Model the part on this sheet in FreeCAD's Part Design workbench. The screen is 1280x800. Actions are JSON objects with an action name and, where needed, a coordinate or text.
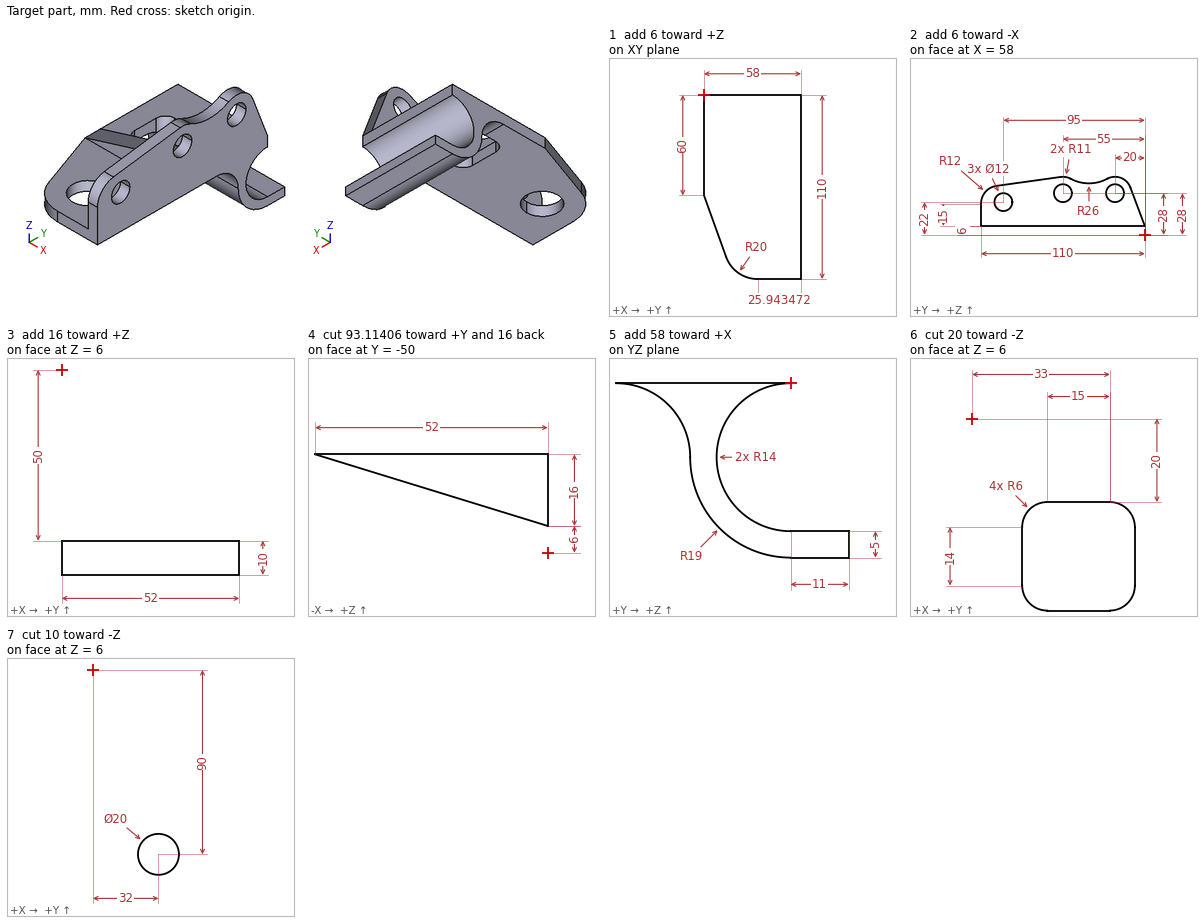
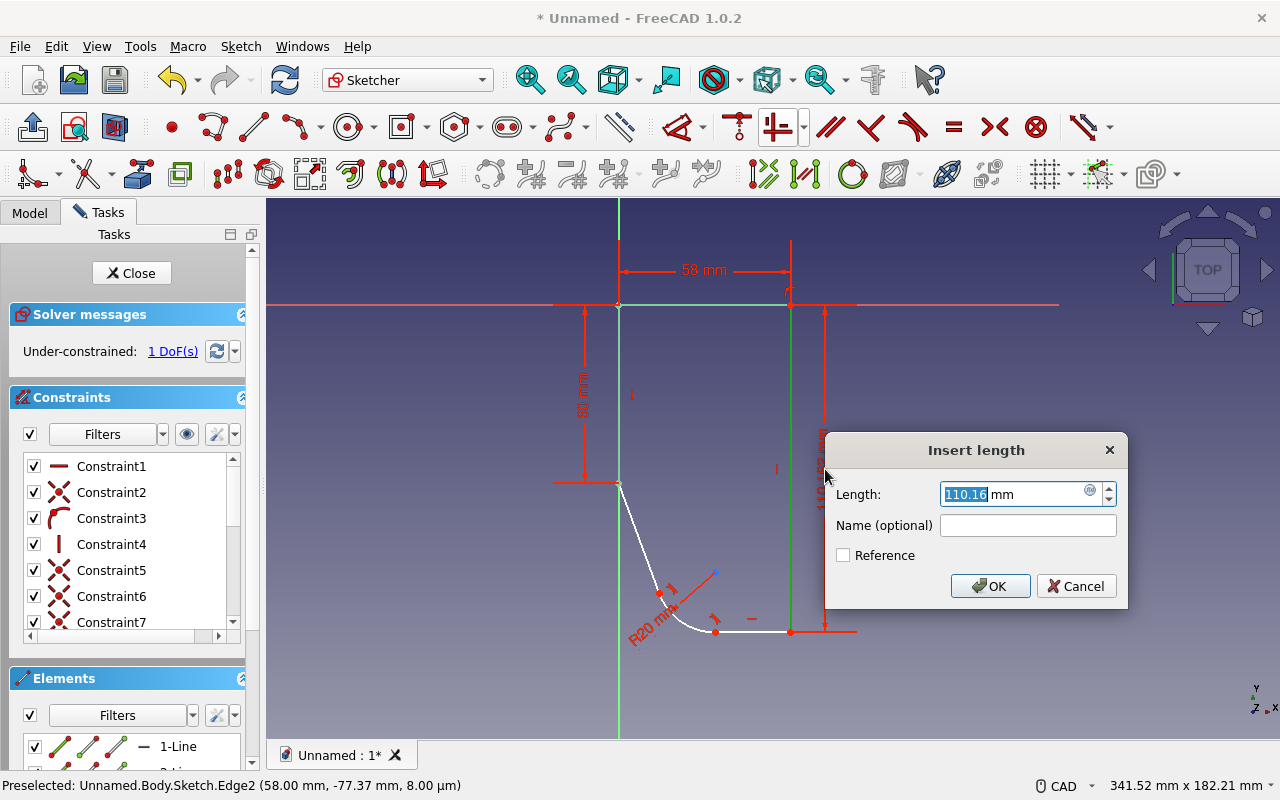
{"action": "type", "text": "110"}
{"action": "key", "text": "Return"}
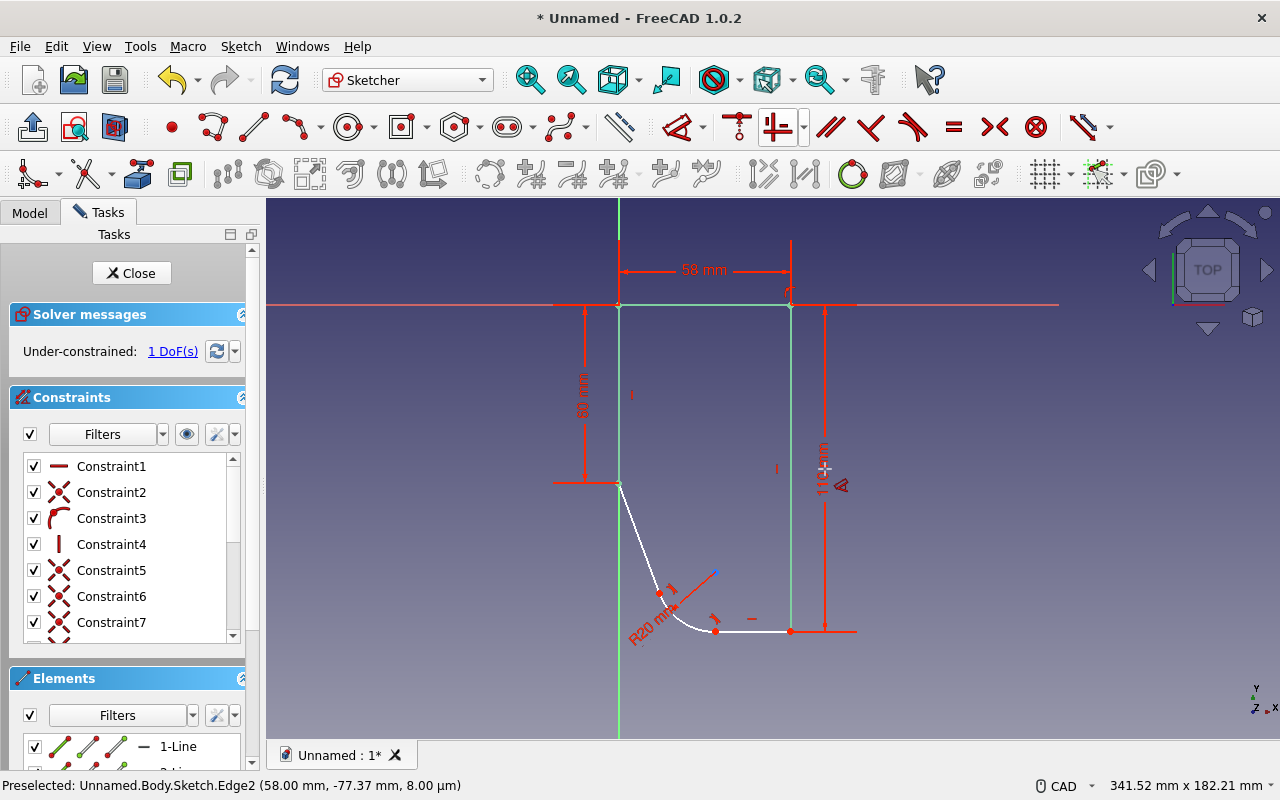
{"action": "left_click", "coordinate": [738, 632]}
{"action": "left_click", "coordinate": [753, 666]}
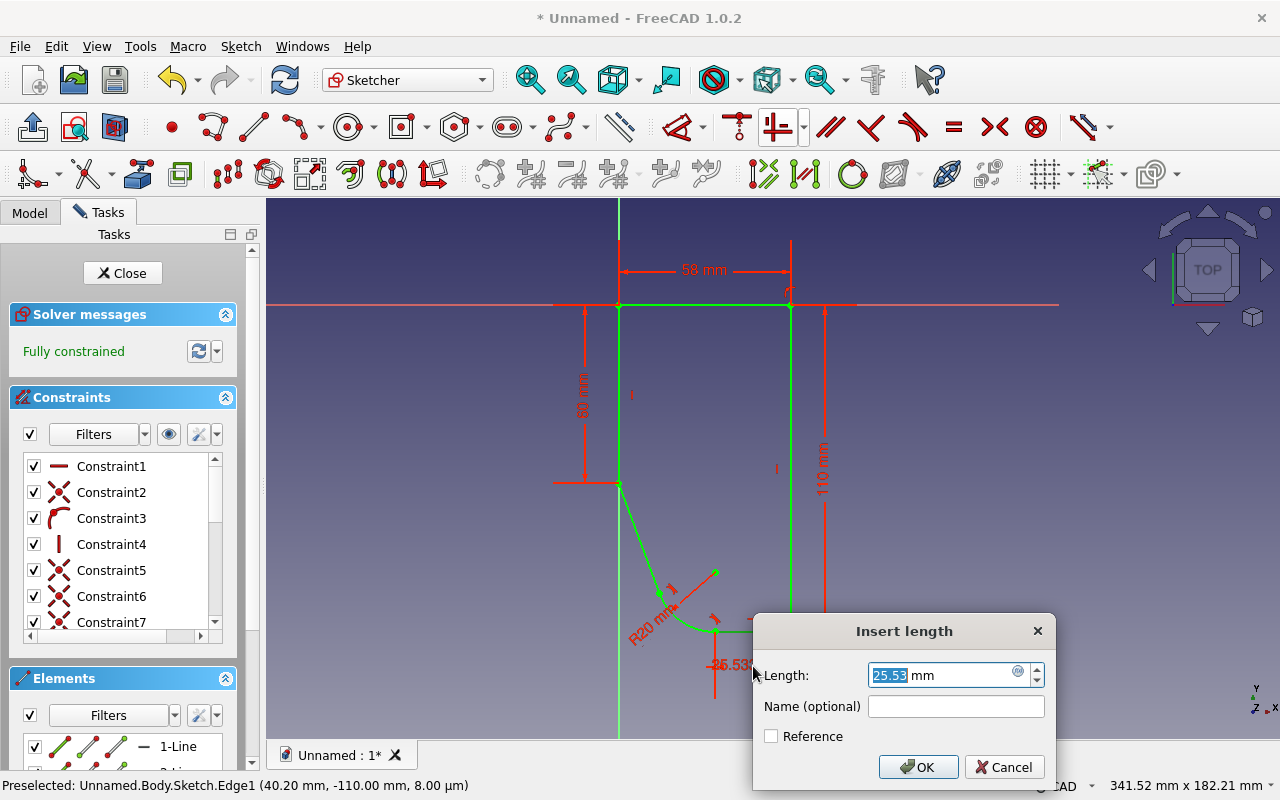
{"action": "type", "text": "25.943472"}
{"action": "key", "text": "Return"}
{"action": "key", "text": "Escape"}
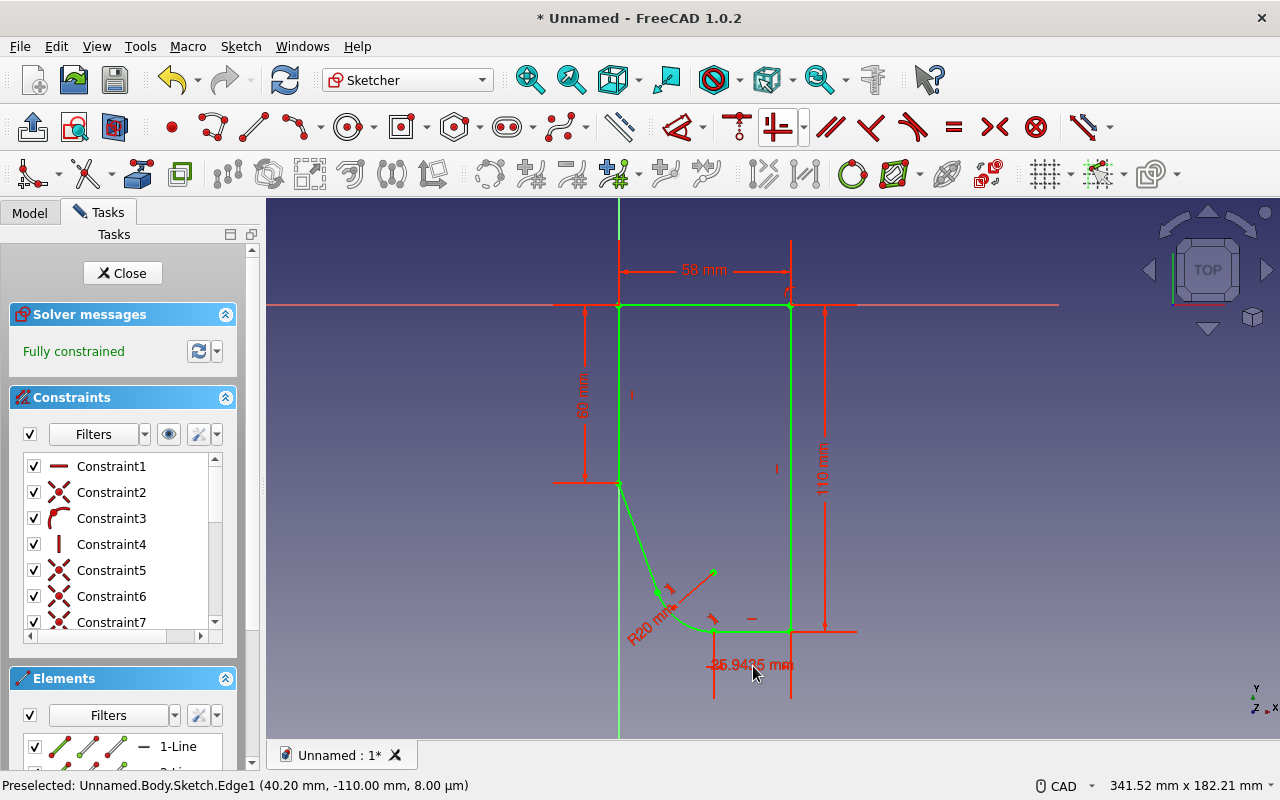
{"action": "left_click", "coordinate": [123, 273]}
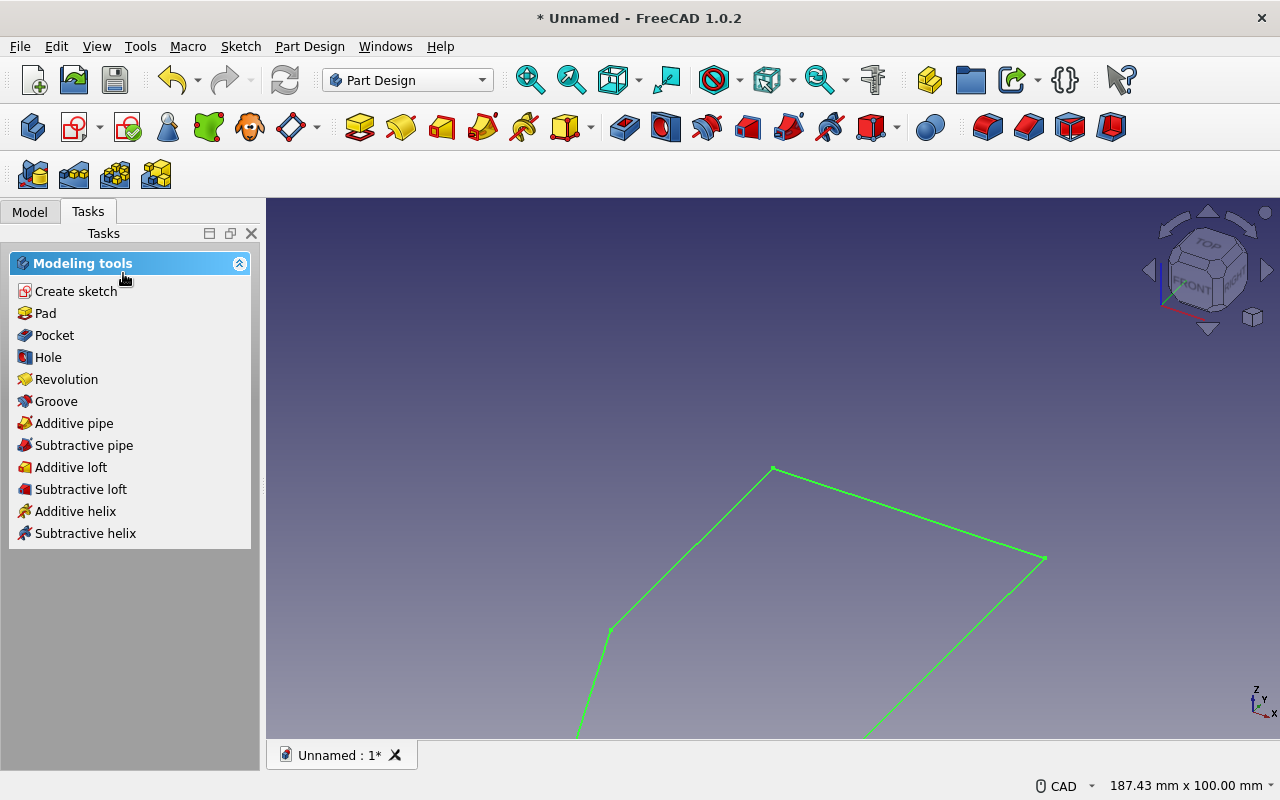
{"action": "left_click", "coordinate": [360, 128]}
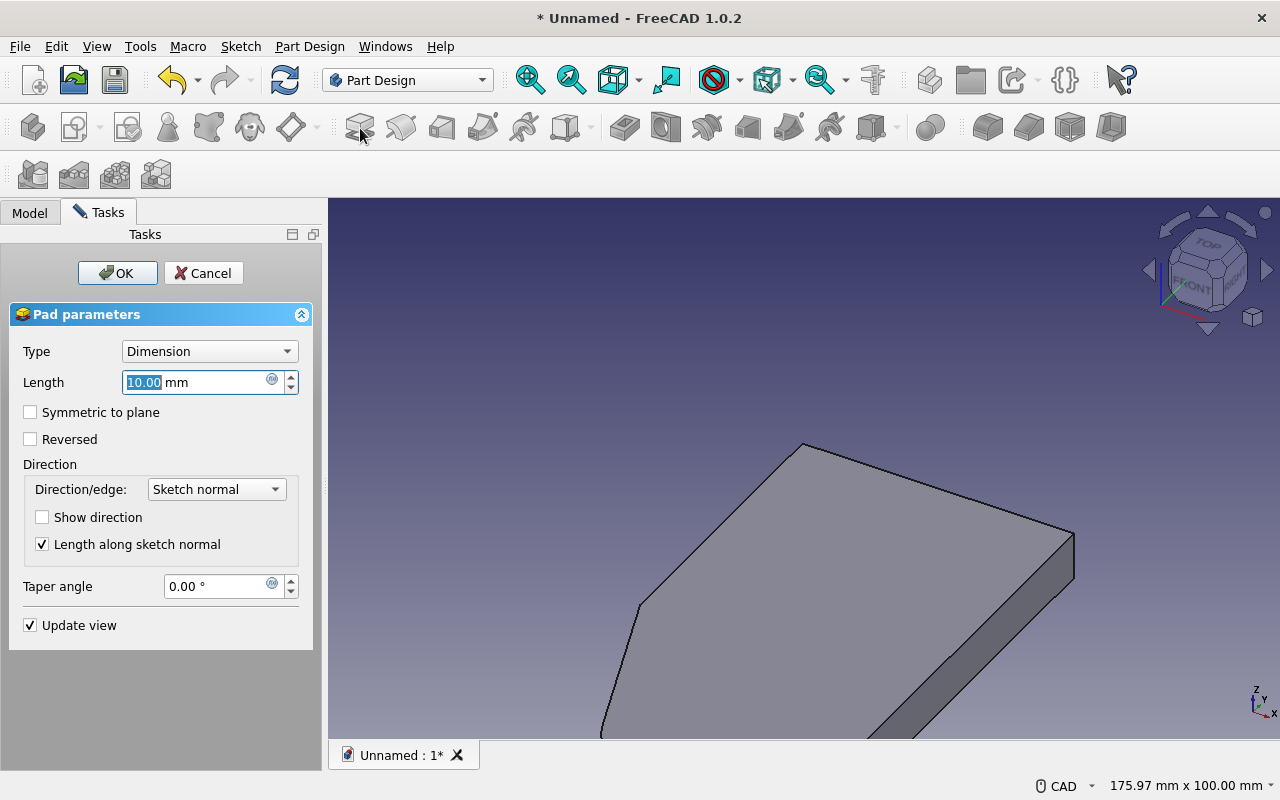
{"action": "type", "text": "6"}
{"action": "key", "text": "Tab"}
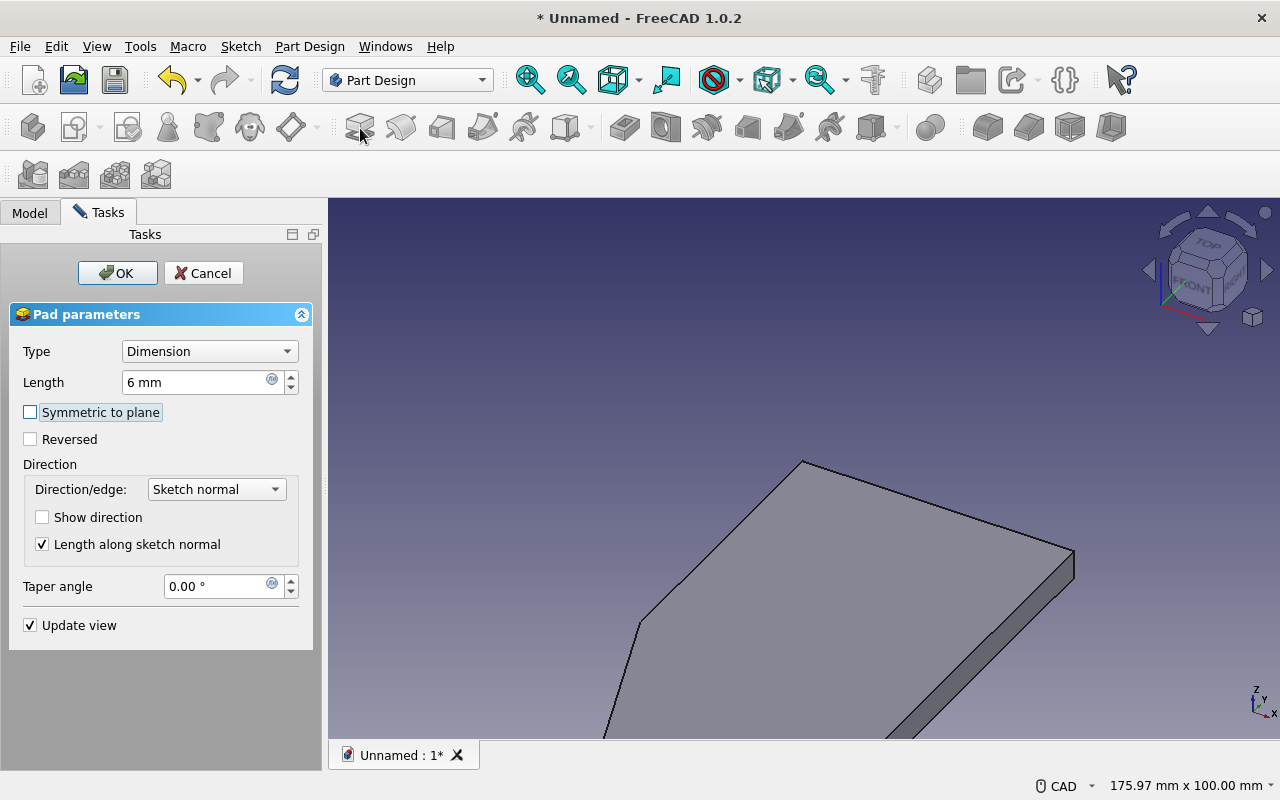
{"action": "left_click", "coordinate": [118, 273]}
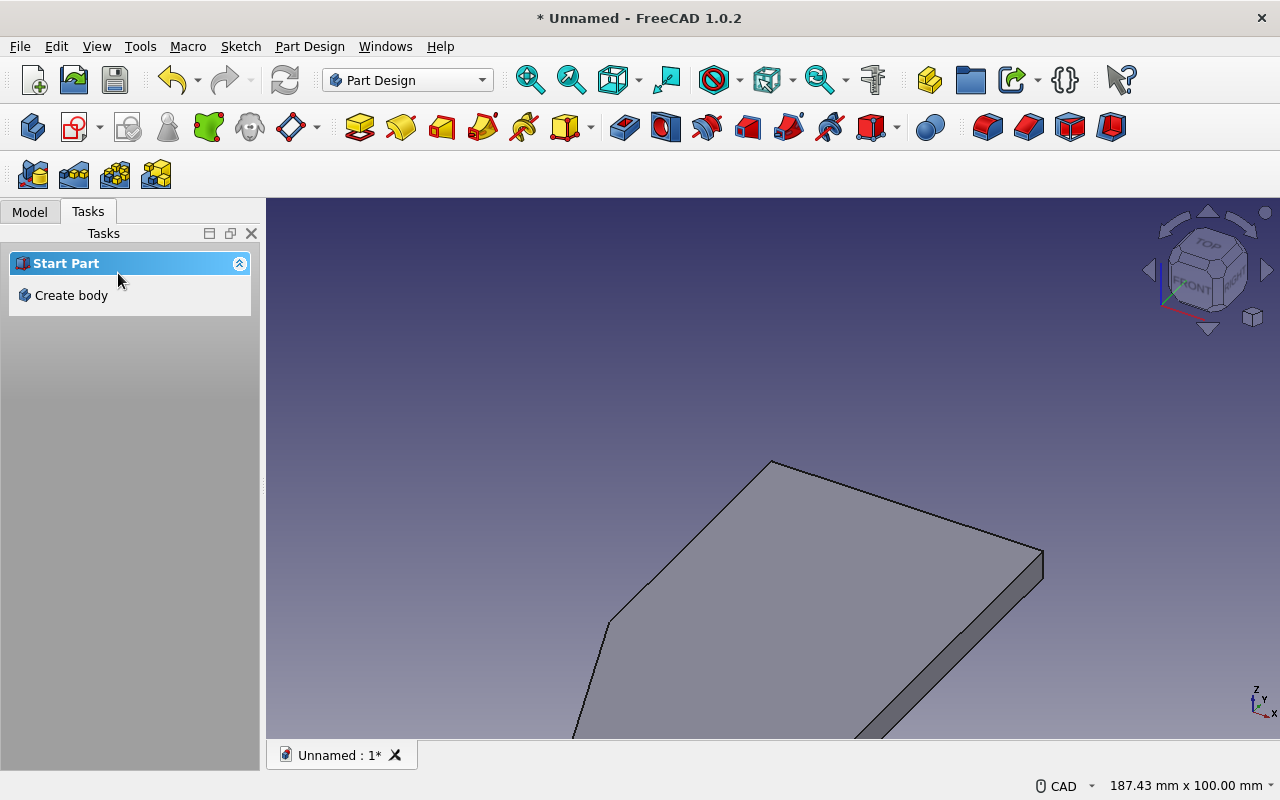
{"action": "left_click", "coordinate": [531, 80]}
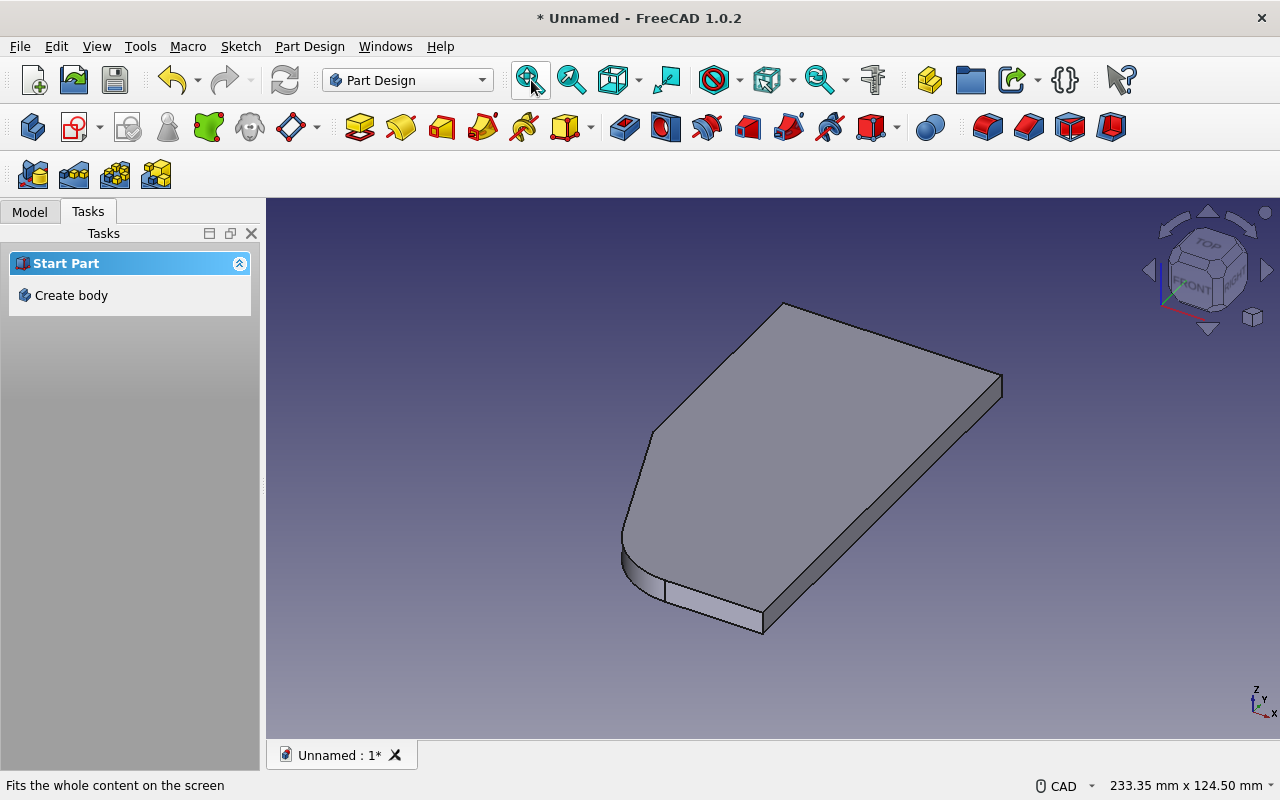
{"action": "key", "text": "0"}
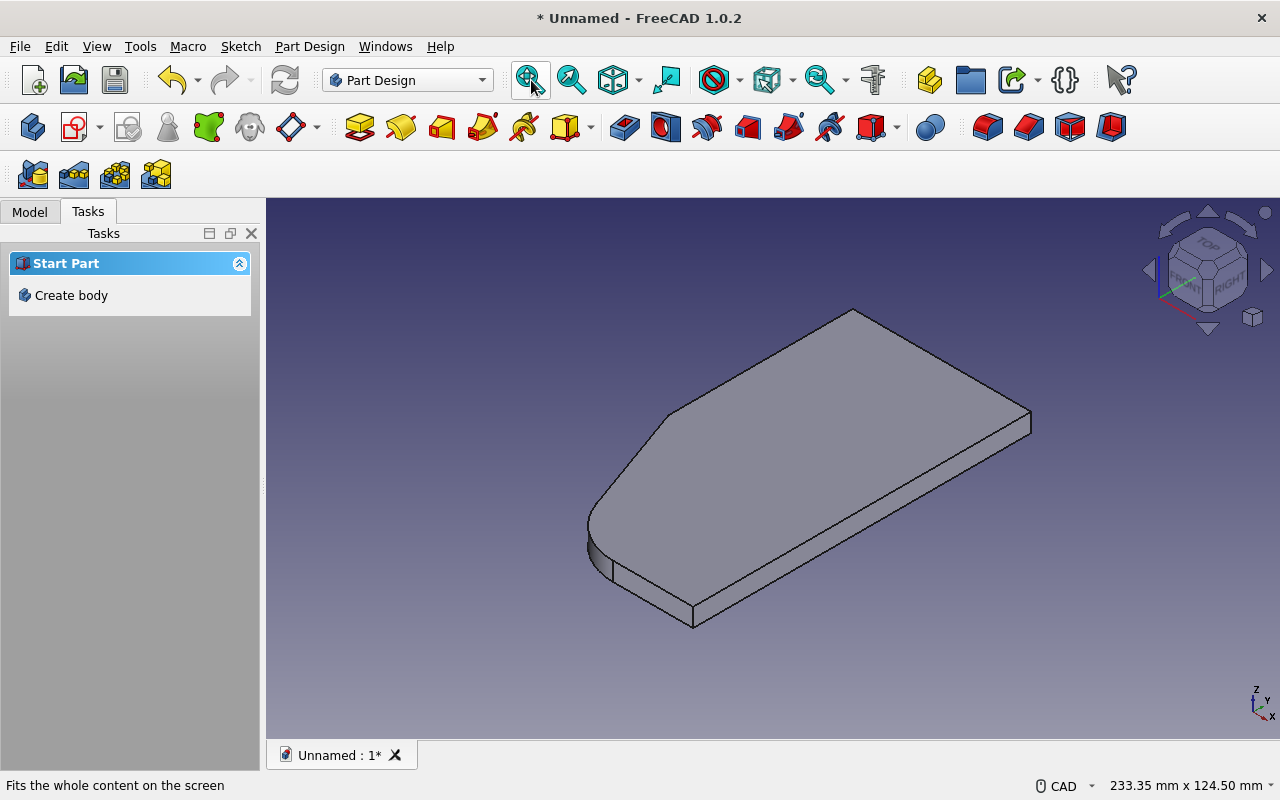
{"action": "left_click", "coordinate": [959, 463]}